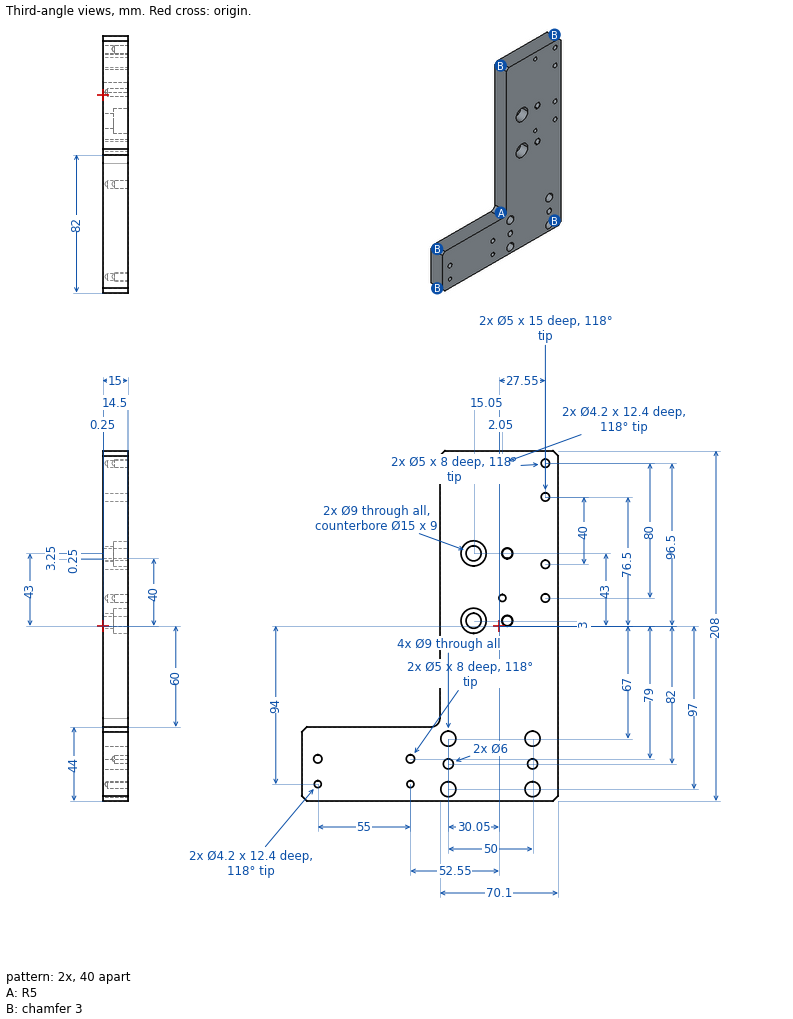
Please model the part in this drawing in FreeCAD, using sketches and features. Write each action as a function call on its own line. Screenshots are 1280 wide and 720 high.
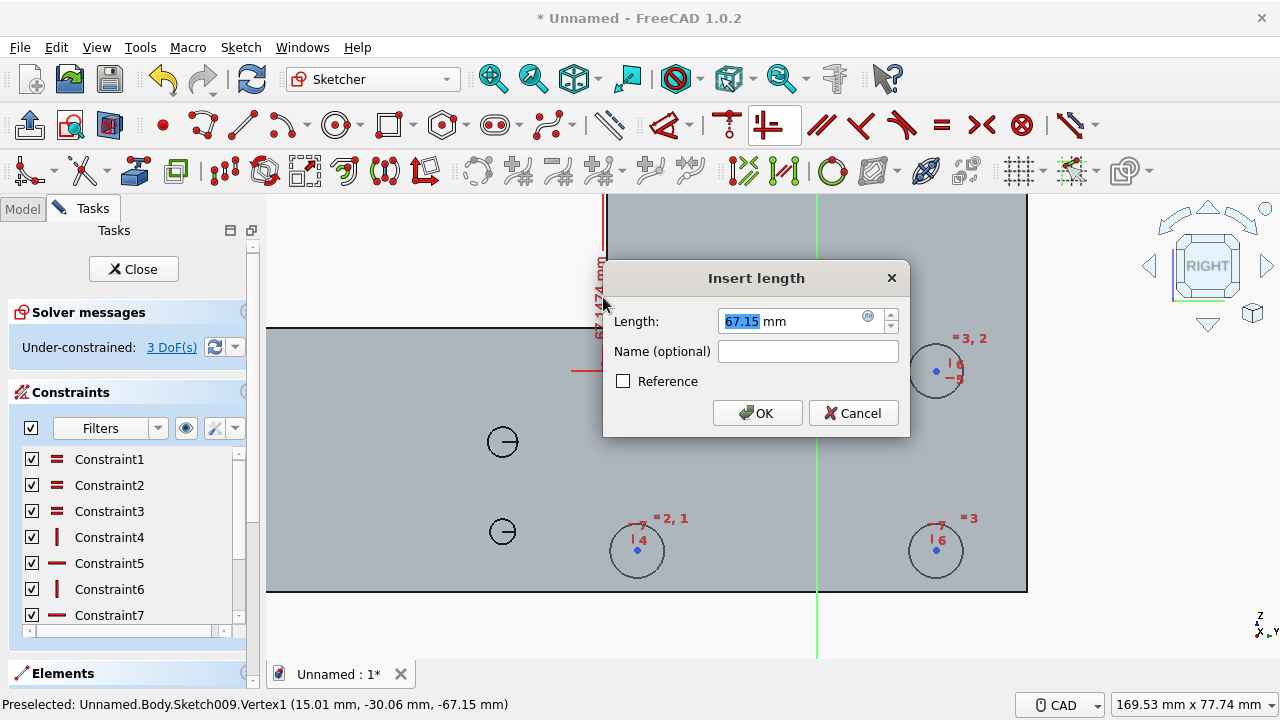
text(67)
key(Return)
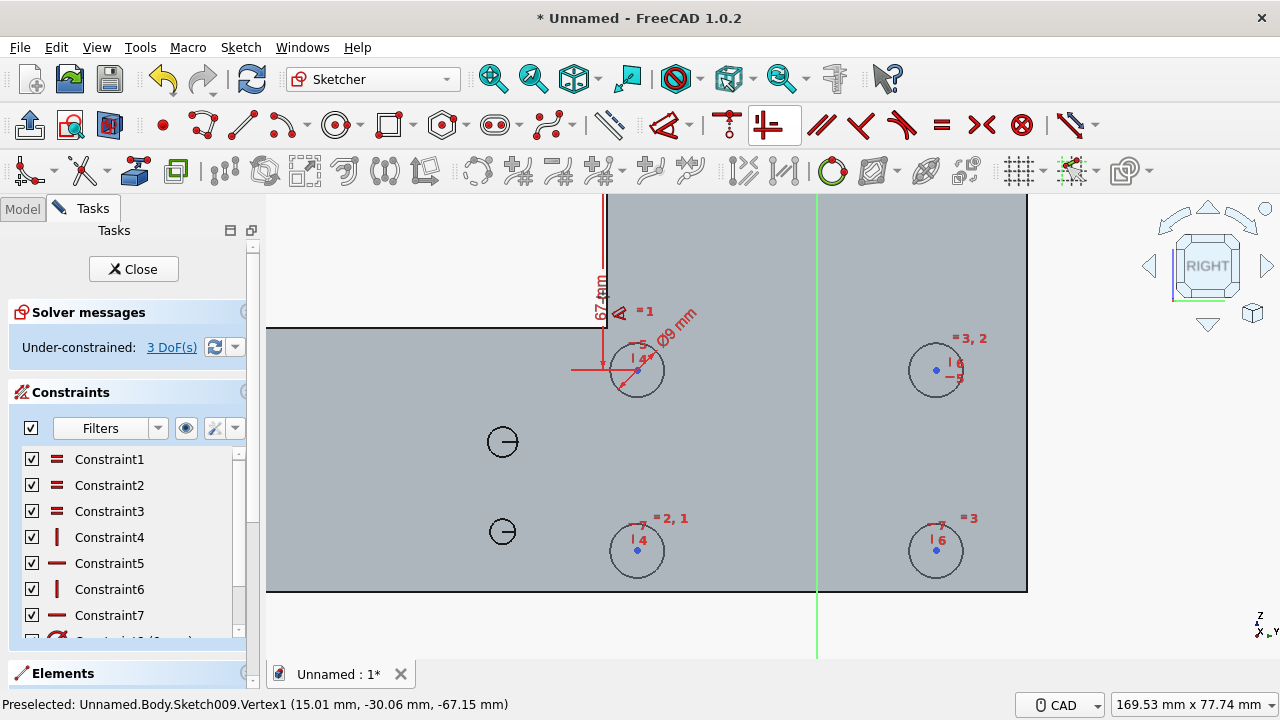
click(637, 551)
click(603, 462)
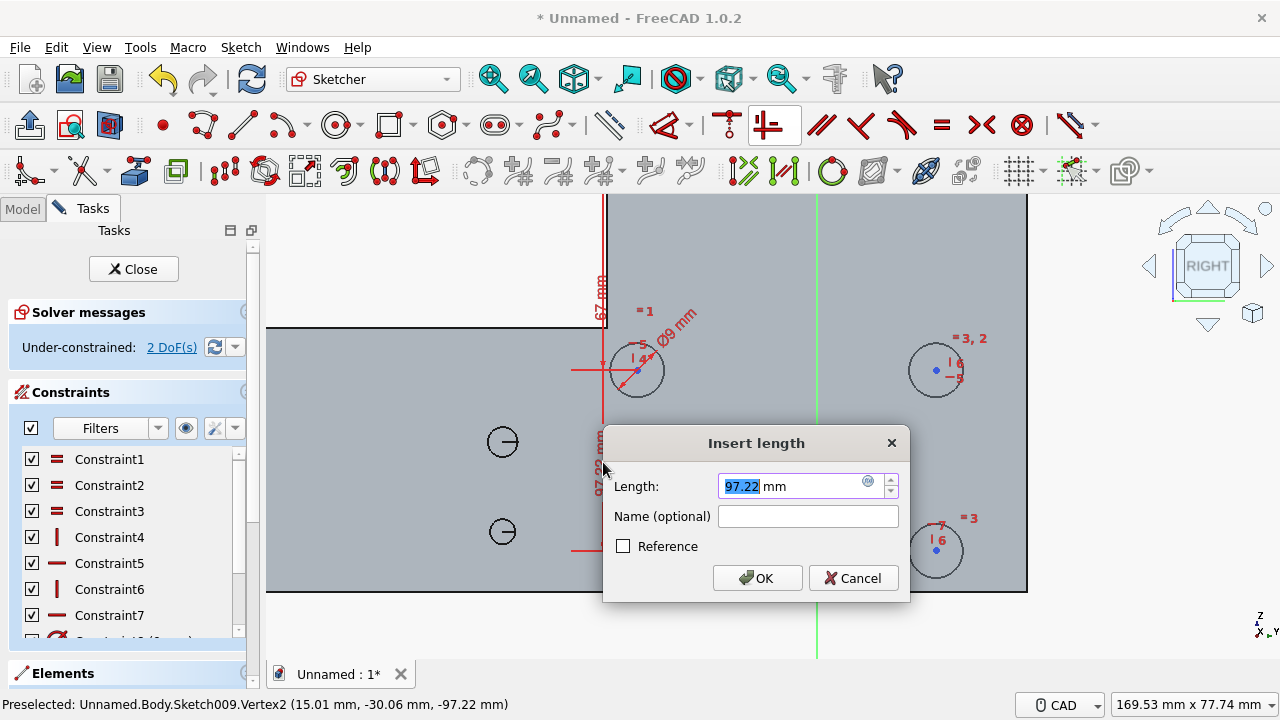
text(97)
key(Return)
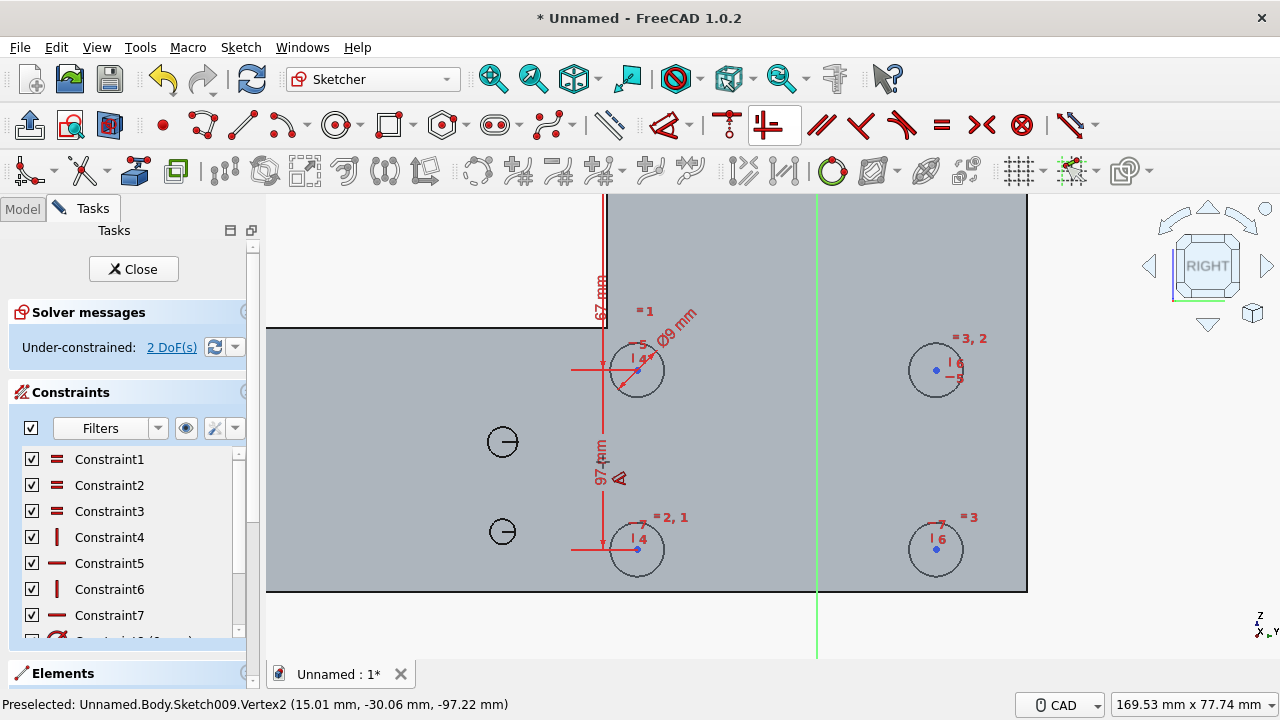
click(637, 370)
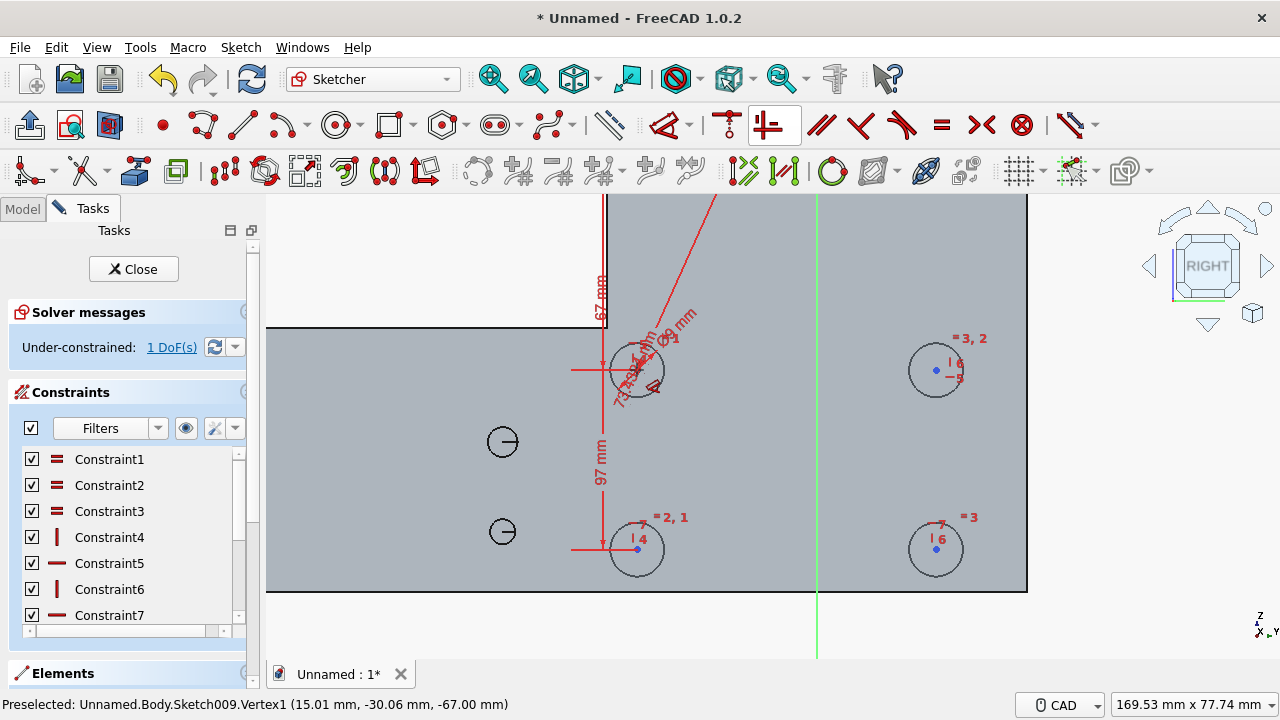
click(936, 370)
click(787, 404)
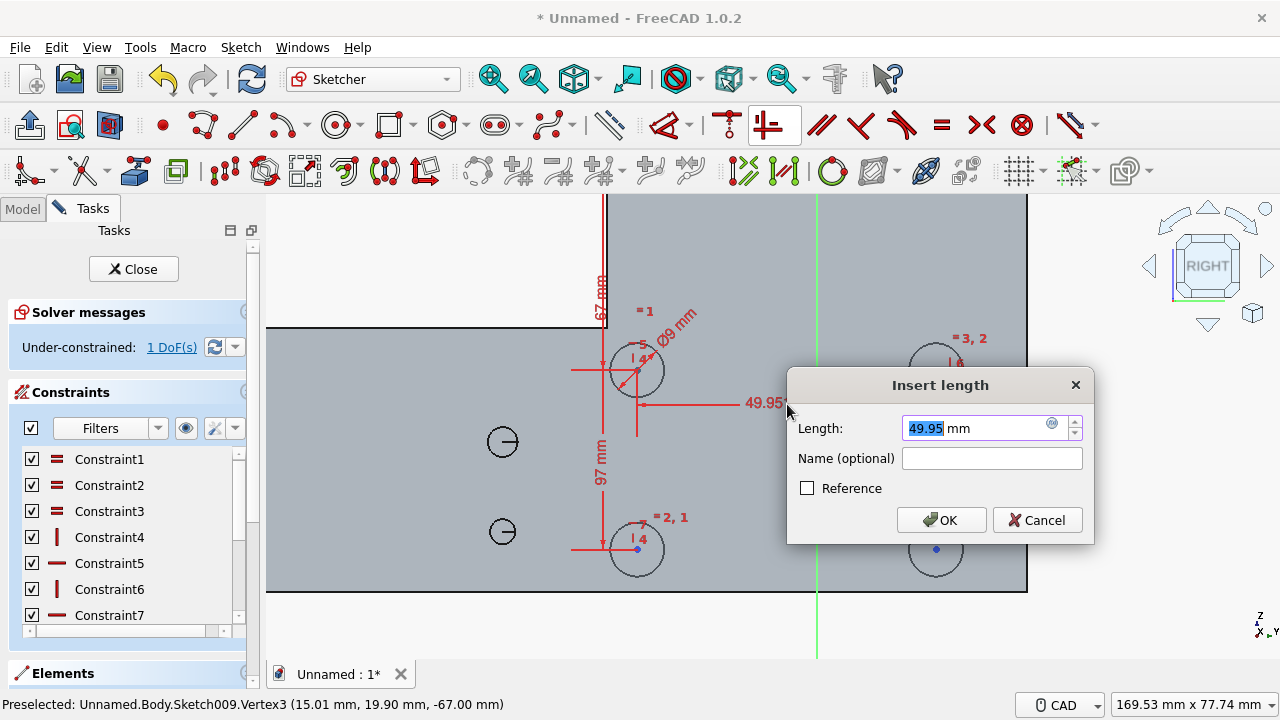
text(50)
key(Return)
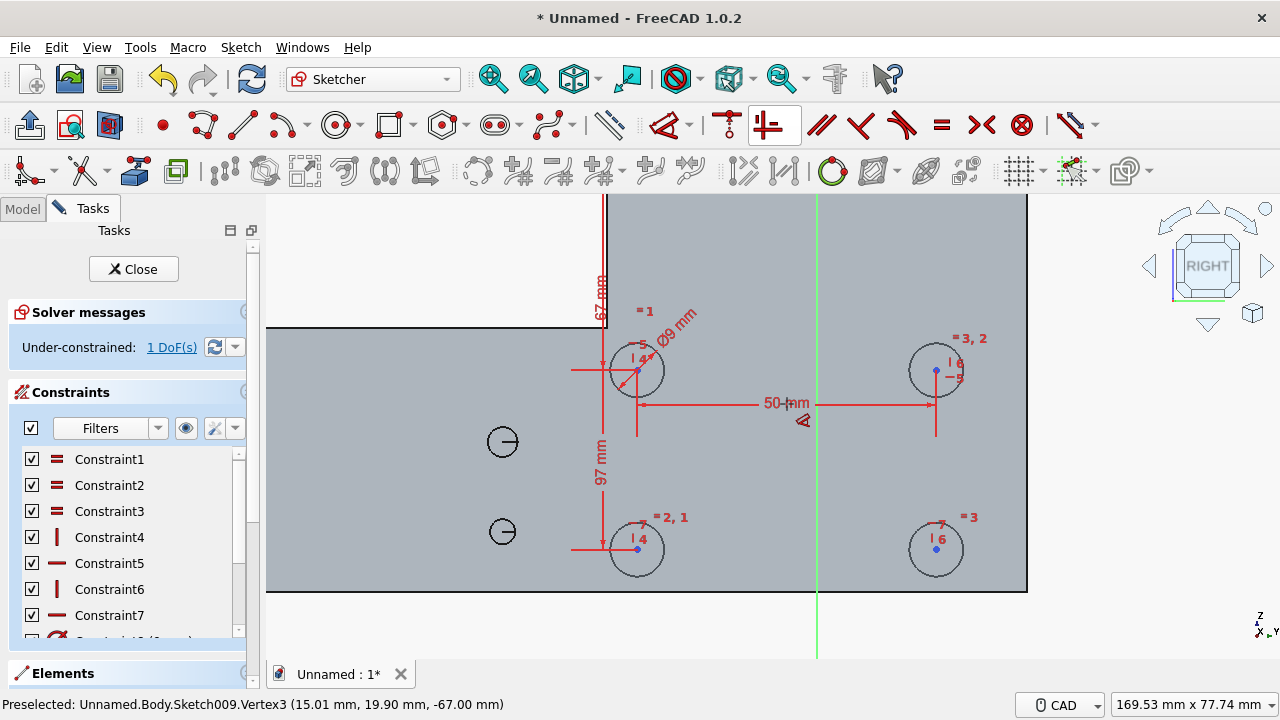
click(637, 370)
click(686, 404)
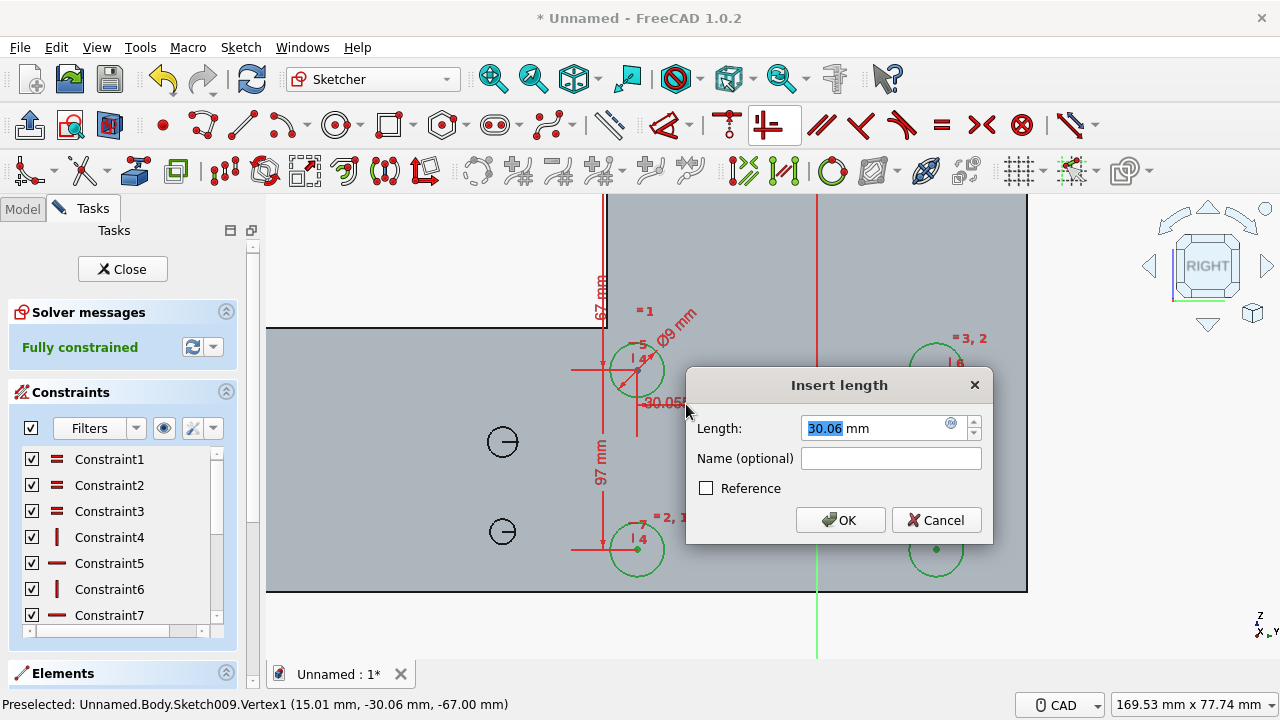
text(30.05)
key(Return)
key(Escape)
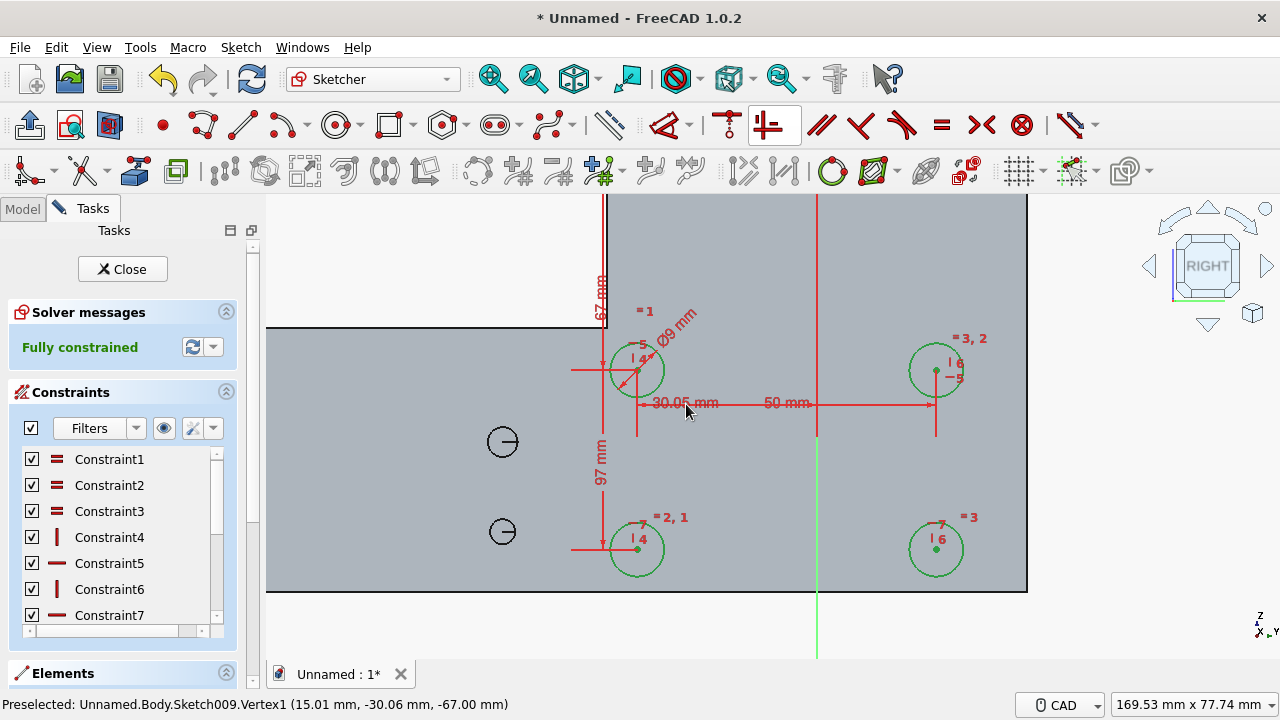
click(123, 269)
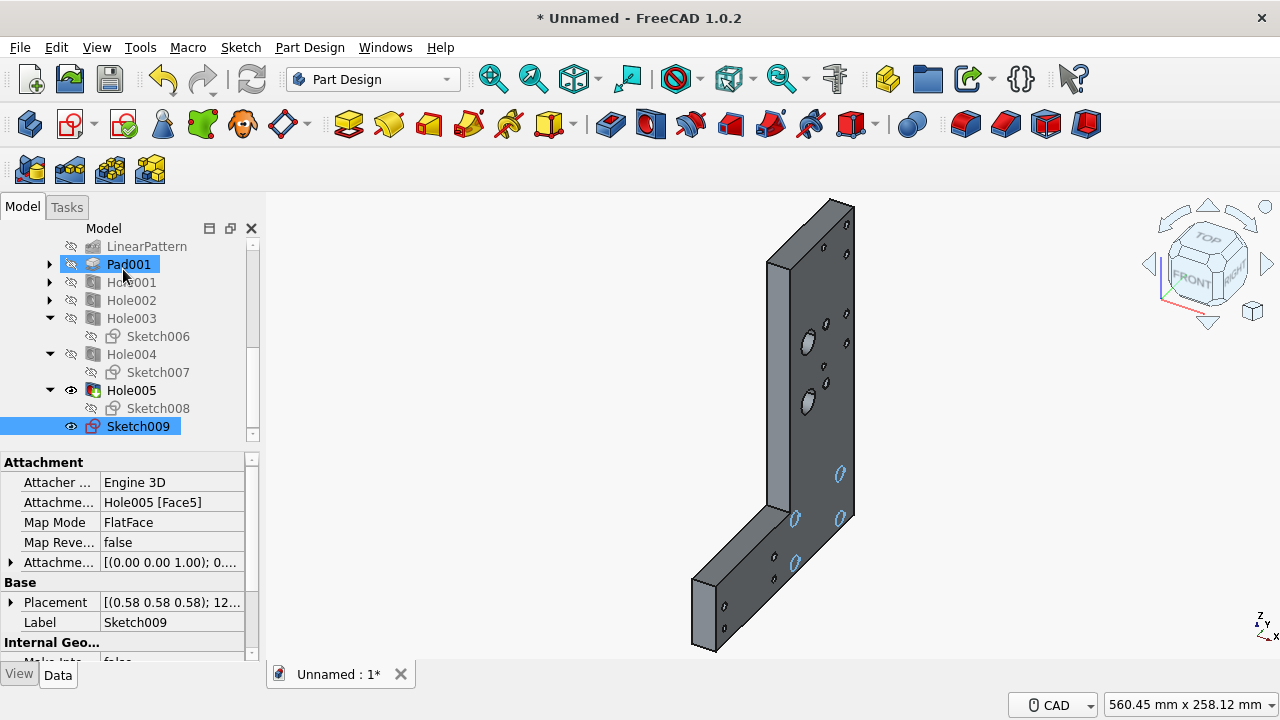
click(652, 124)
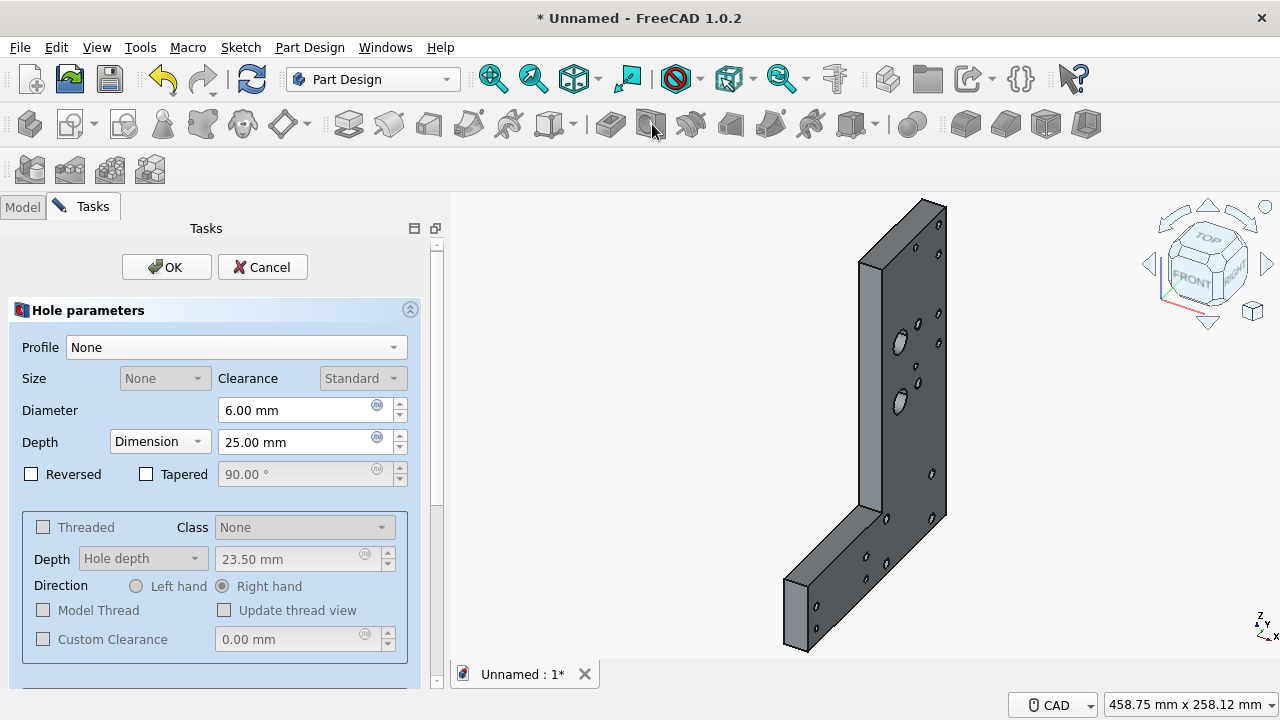
triple_click(305, 410)